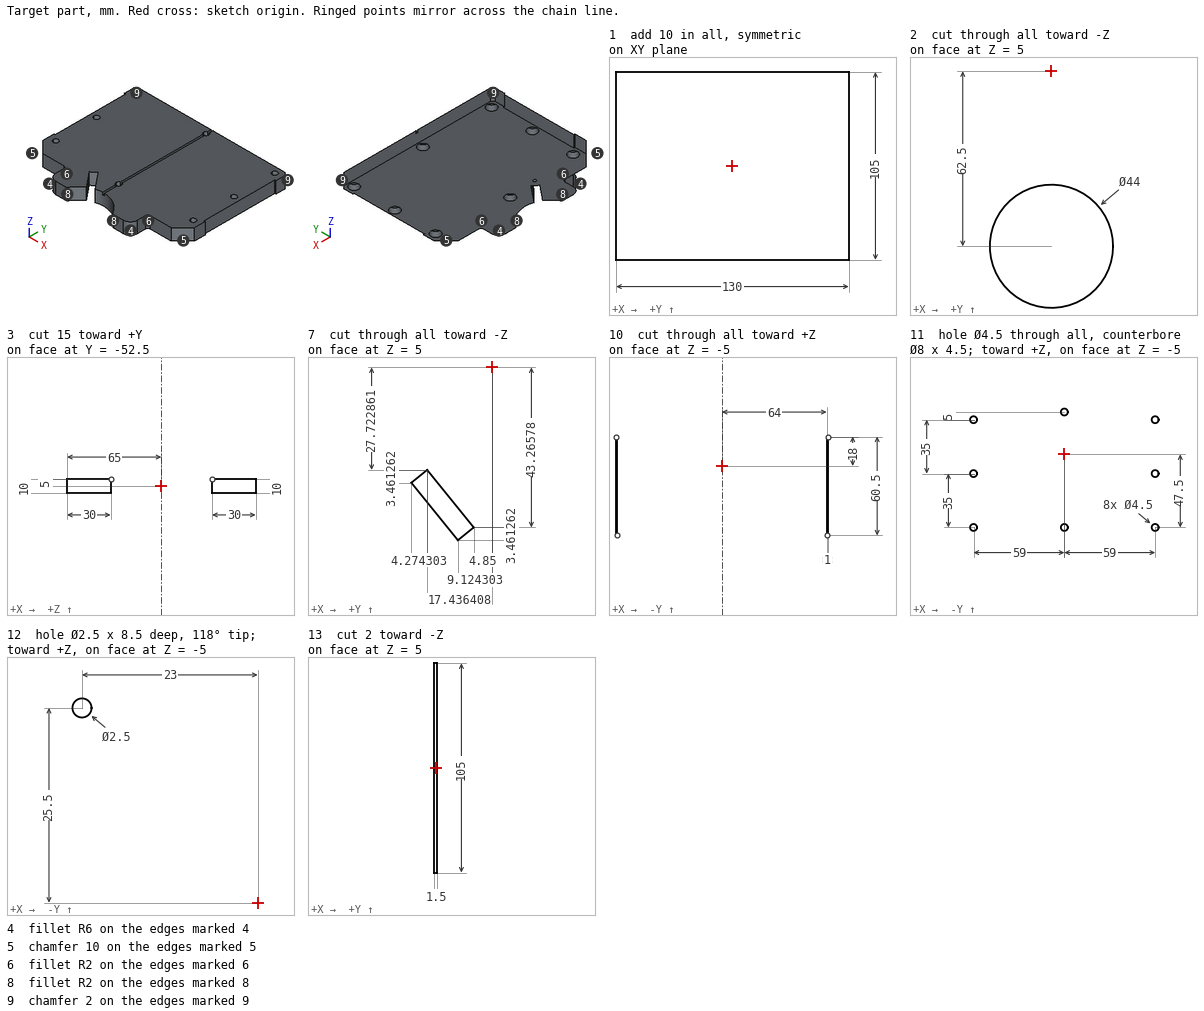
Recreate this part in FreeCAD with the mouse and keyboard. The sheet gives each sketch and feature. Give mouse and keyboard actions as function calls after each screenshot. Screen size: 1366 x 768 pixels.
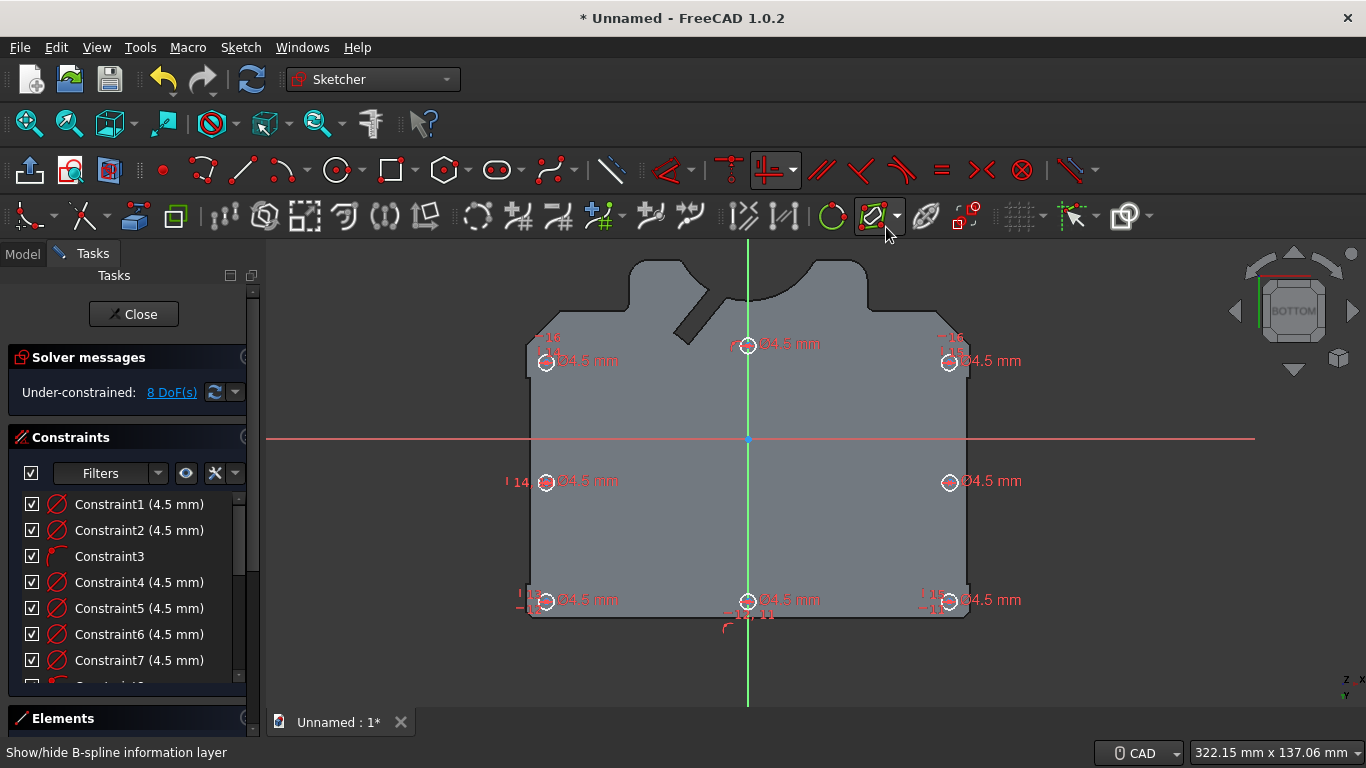
click(949, 602)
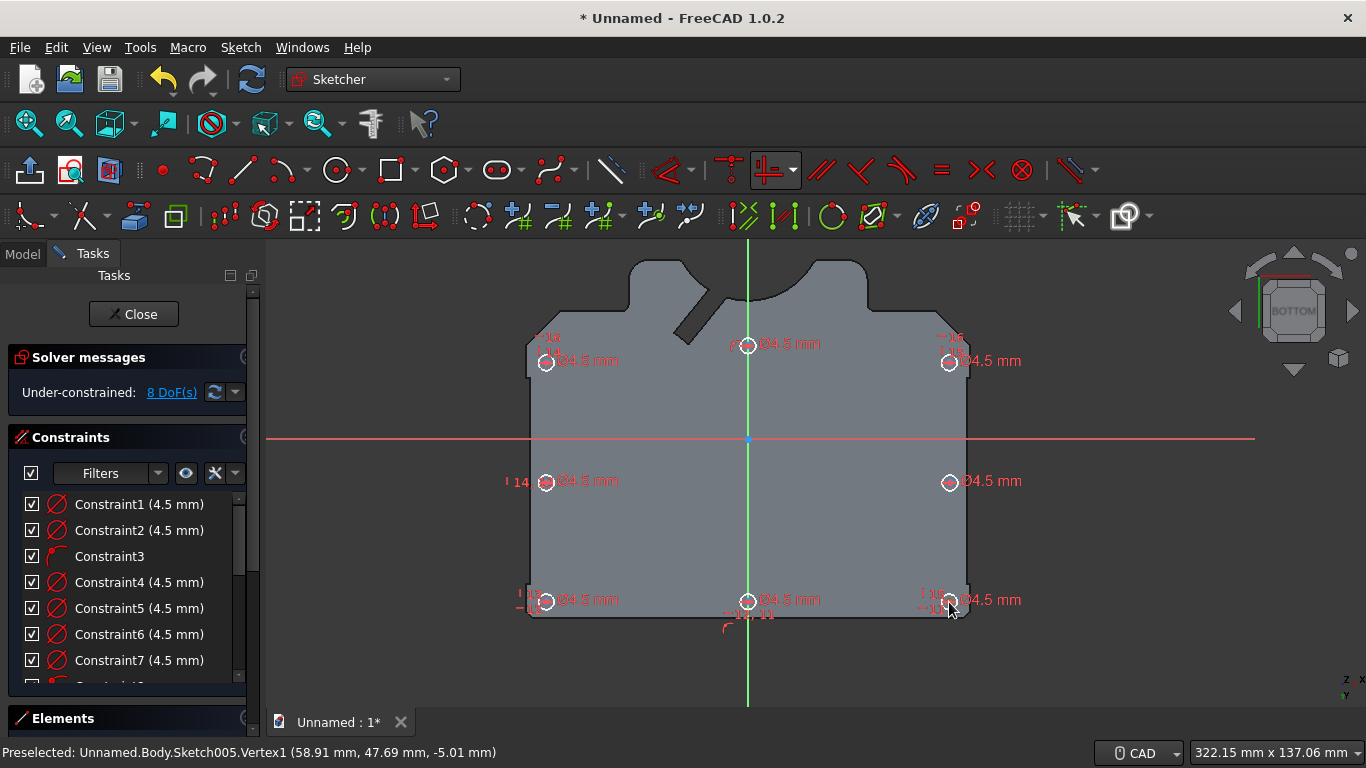
click(950, 483)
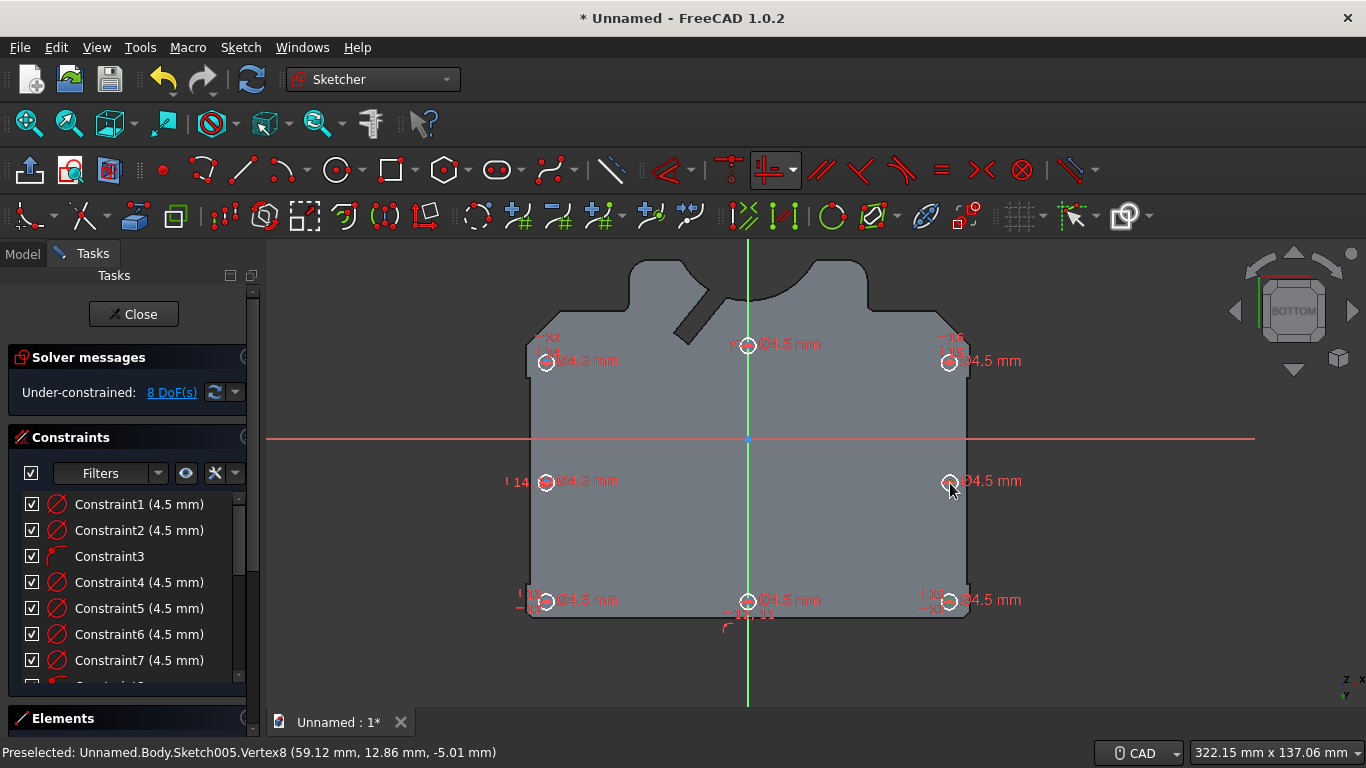
click(796, 170)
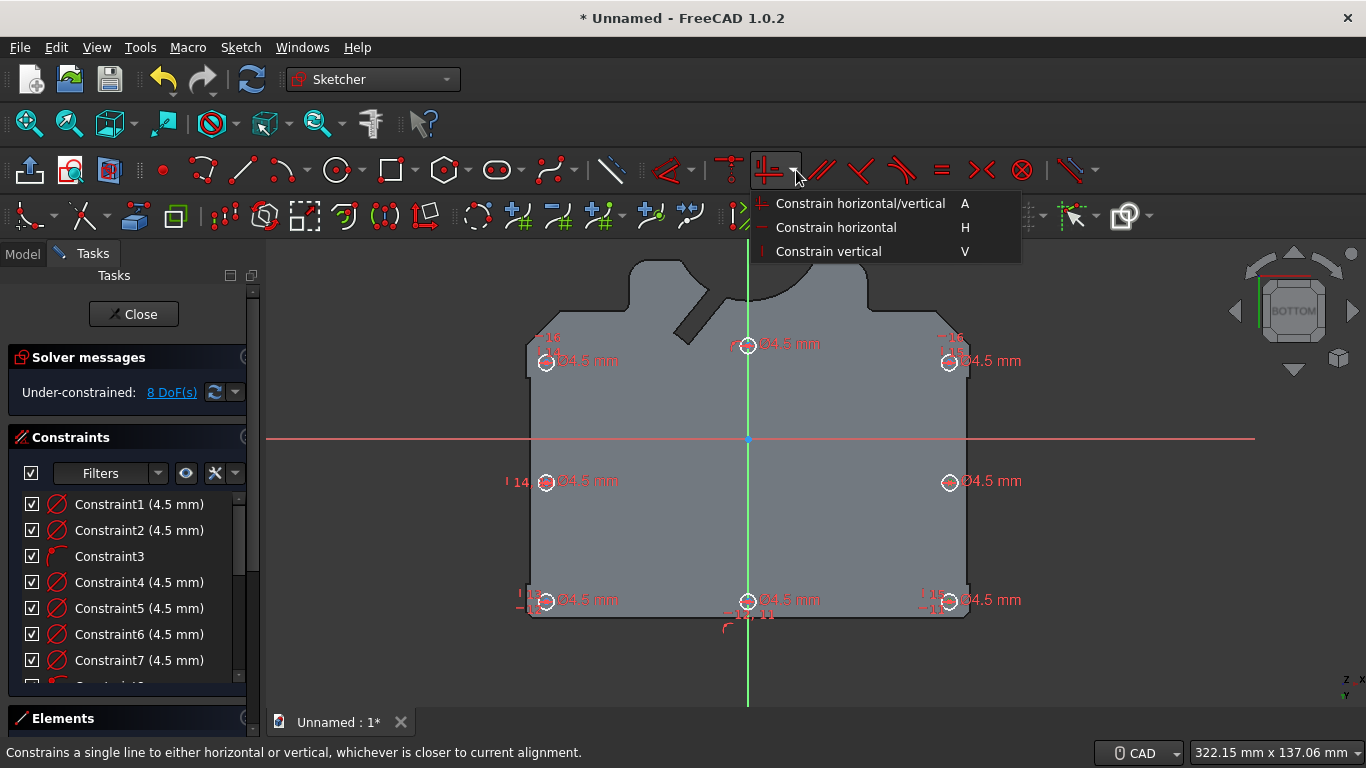
click(886, 251)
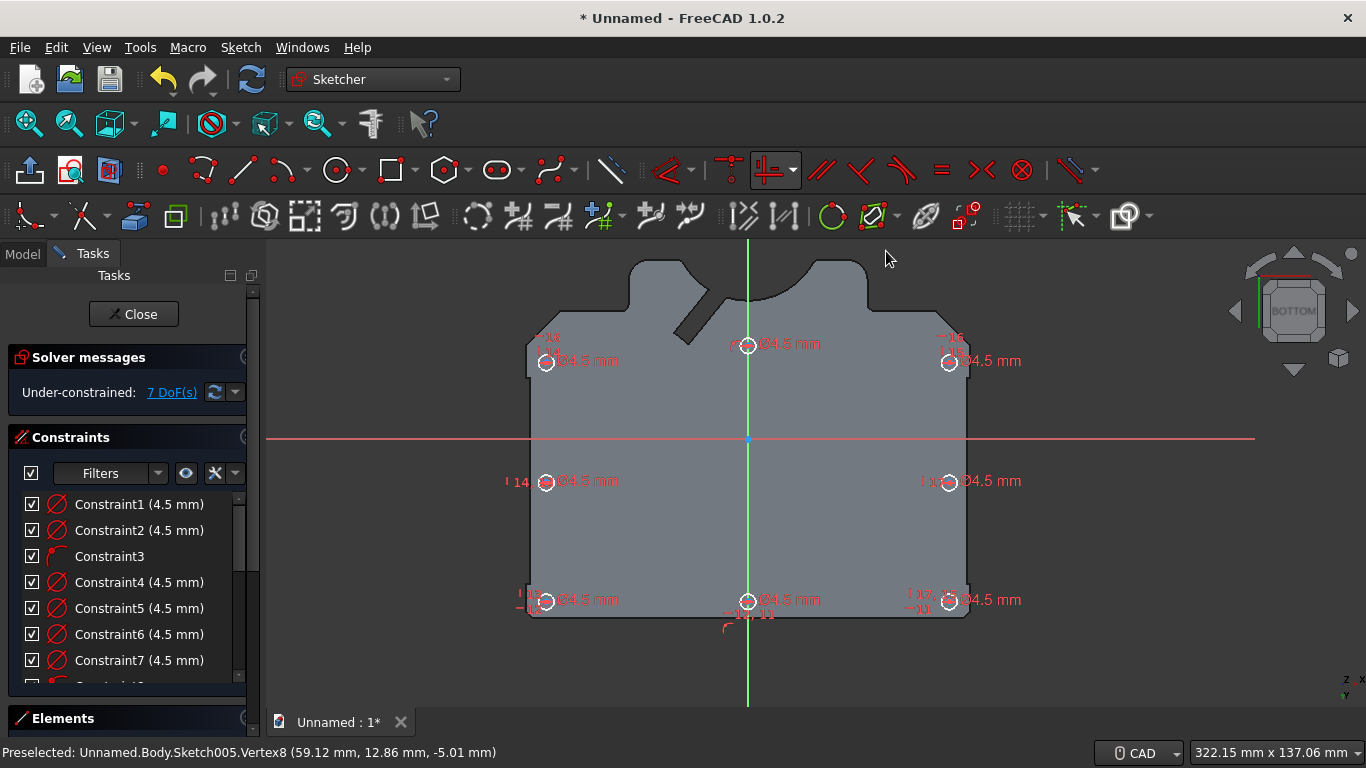
click(546, 483)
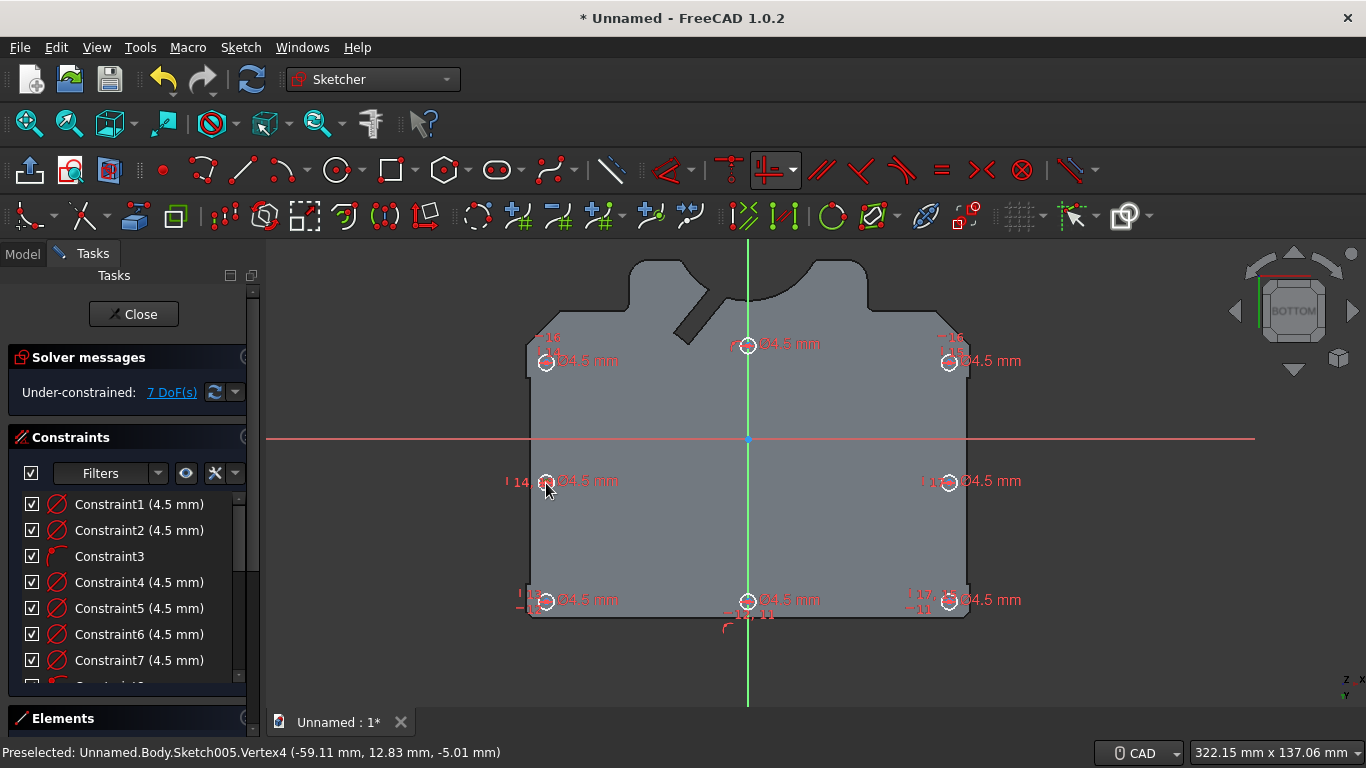
click(949, 483)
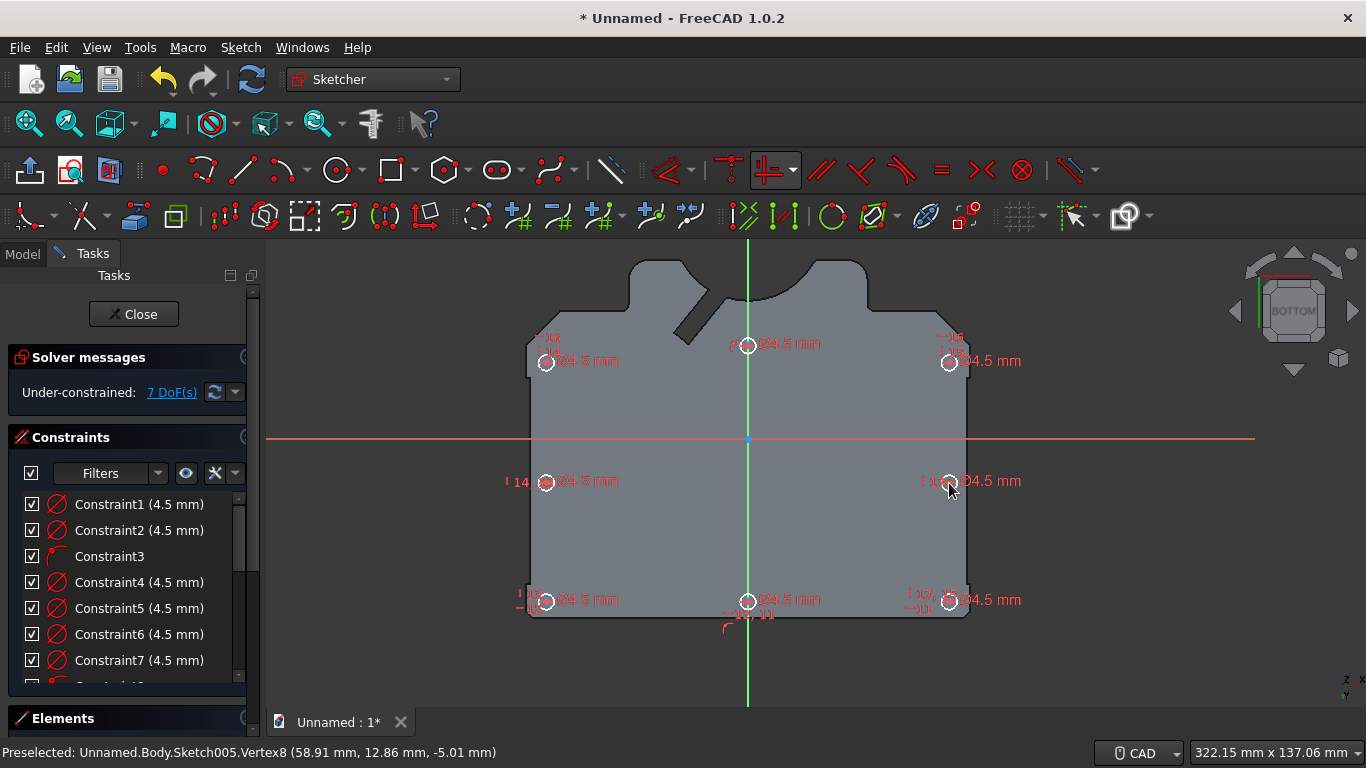
key(h)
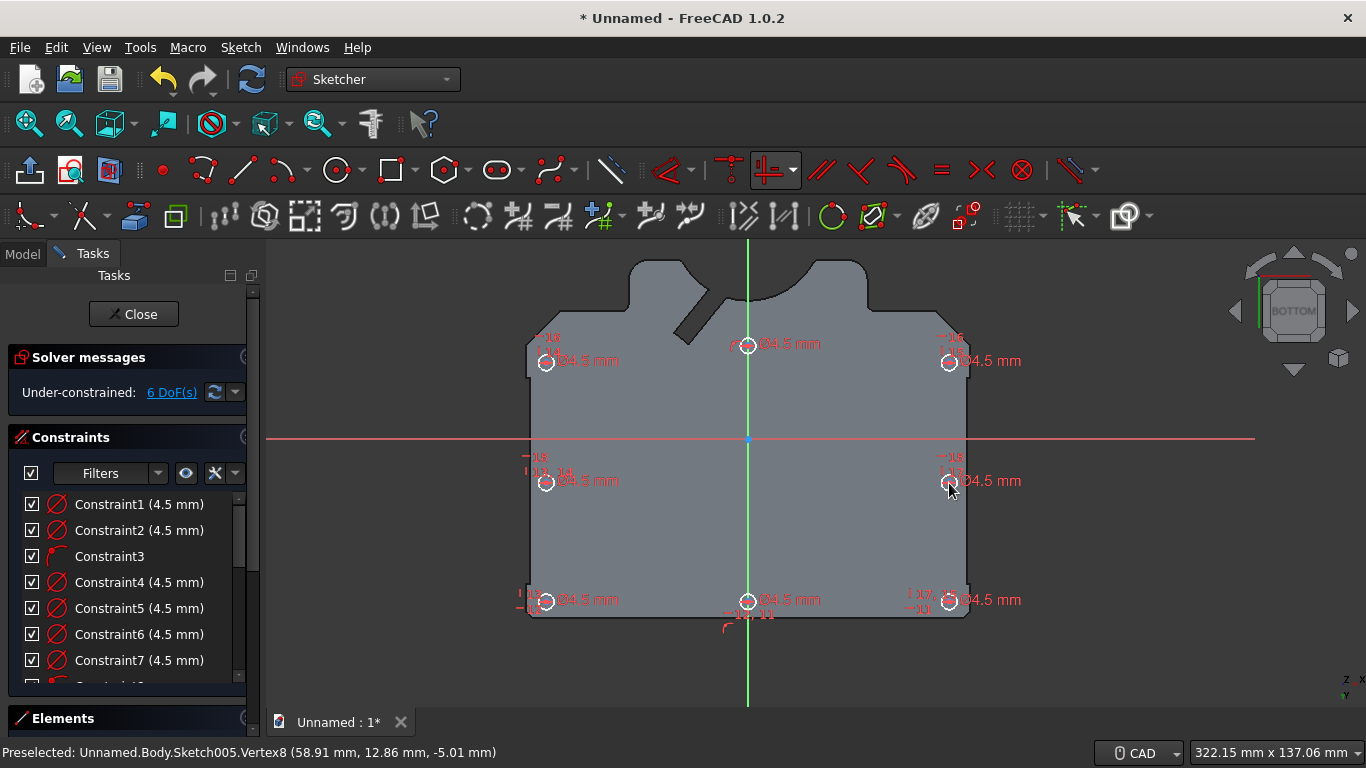
click(666, 170)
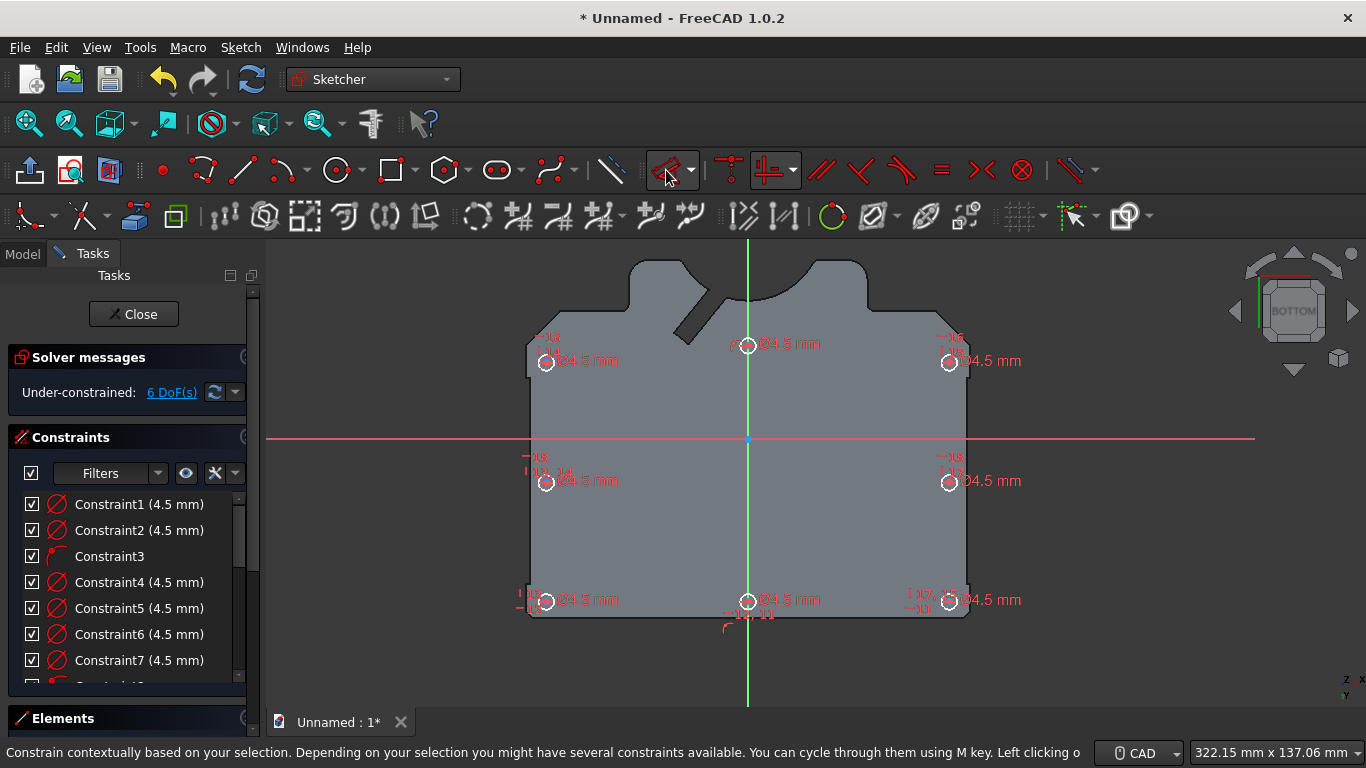
click(949, 602)
click(849, 636)